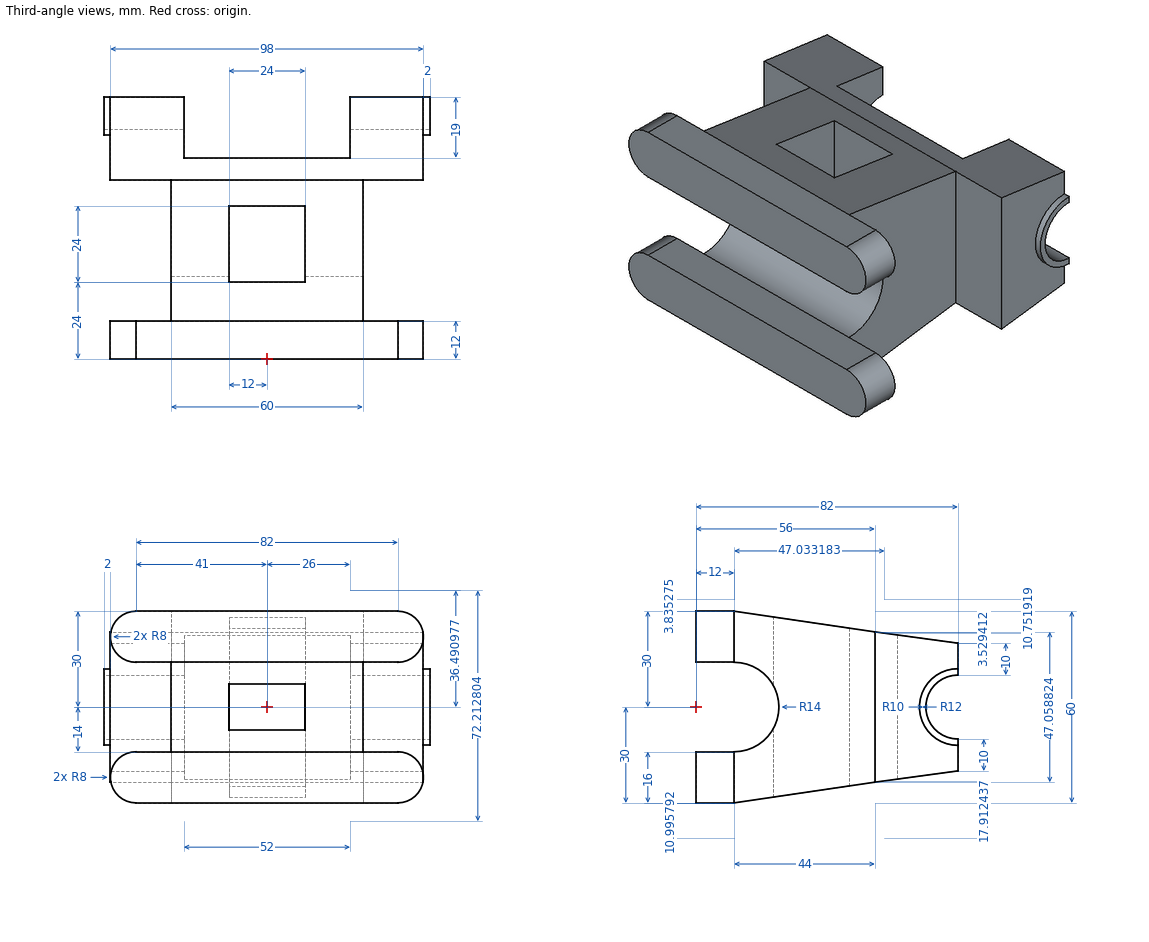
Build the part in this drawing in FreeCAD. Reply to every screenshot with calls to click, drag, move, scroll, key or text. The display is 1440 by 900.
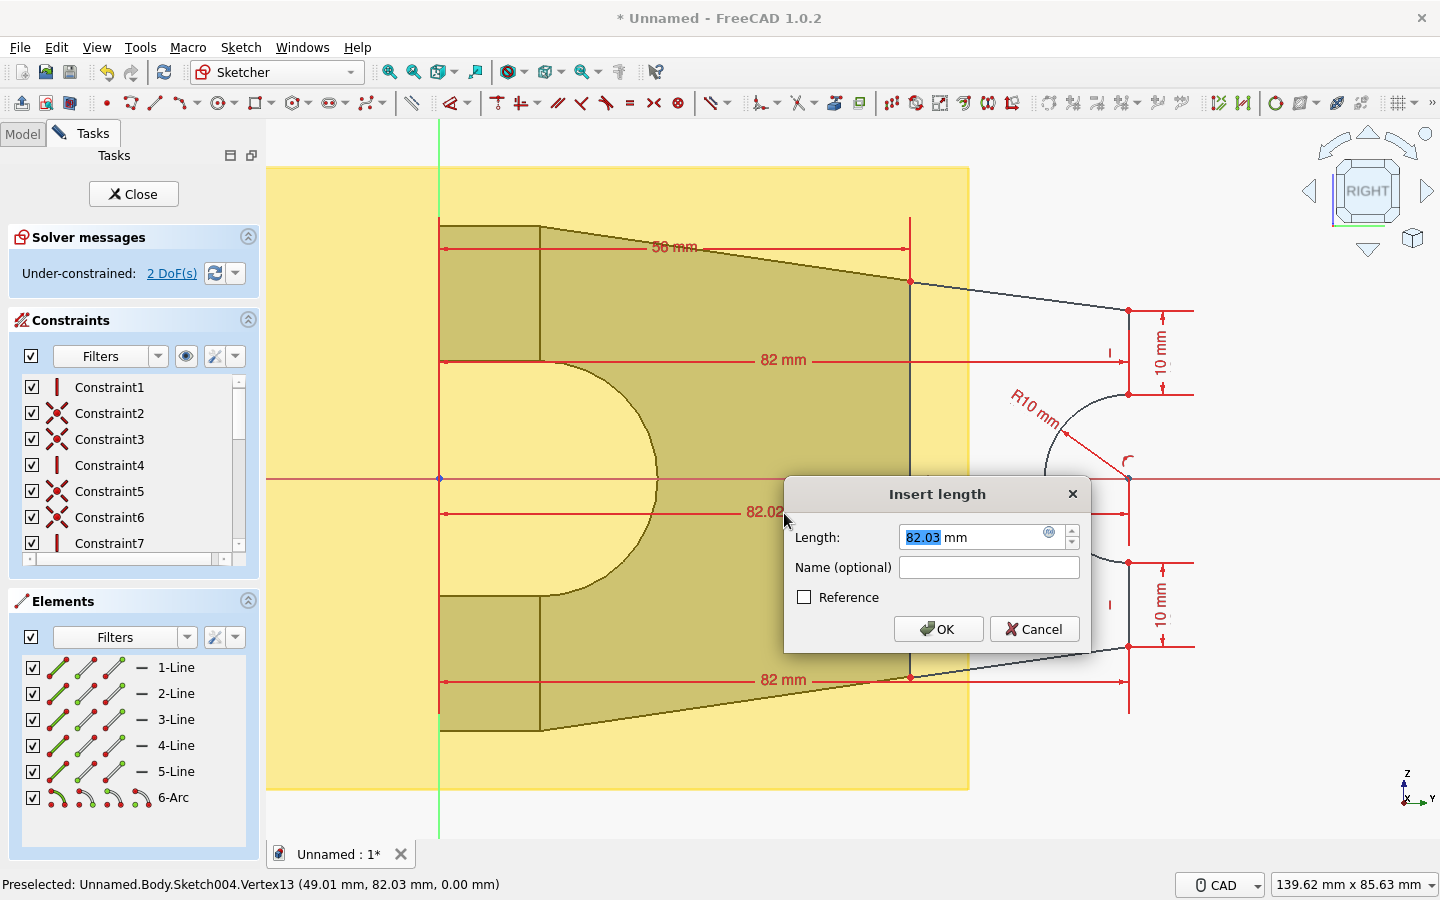
text(82)
key(Return)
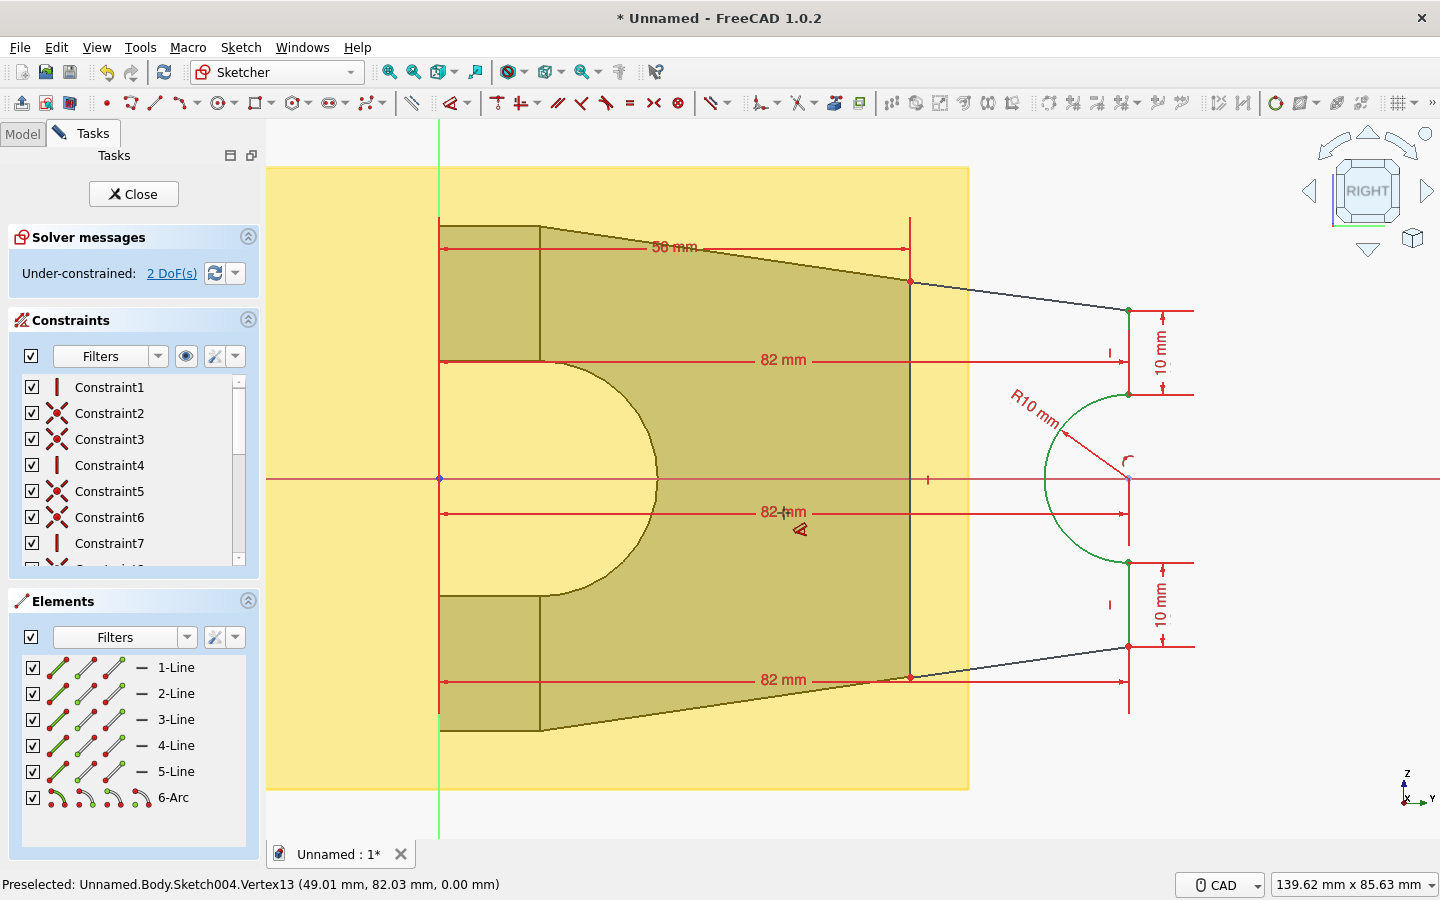
click(910, 401)
click(944, 389)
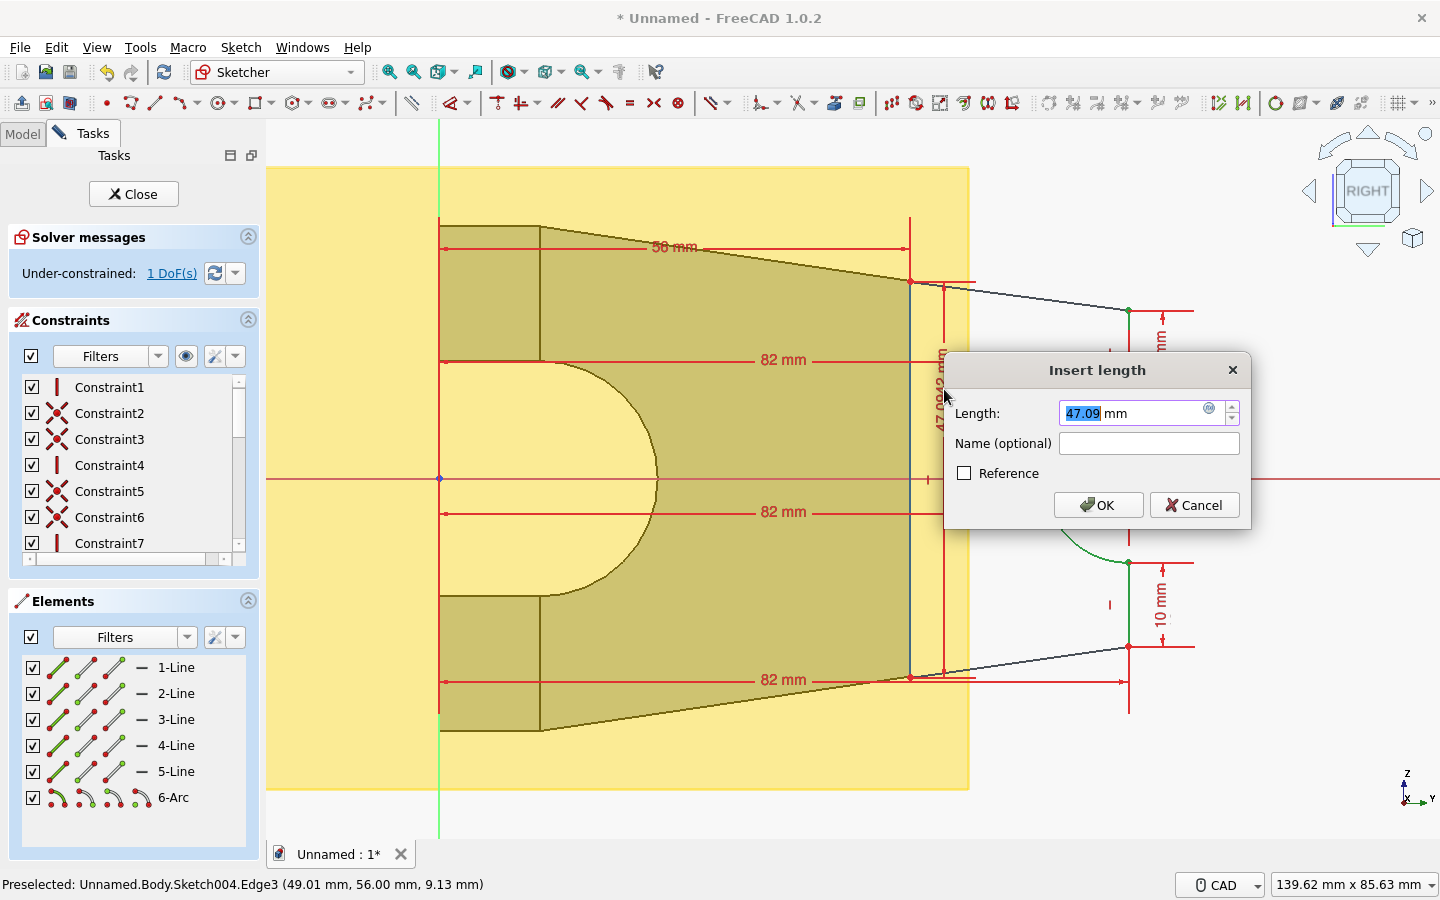
text(47.058824)
key(Return)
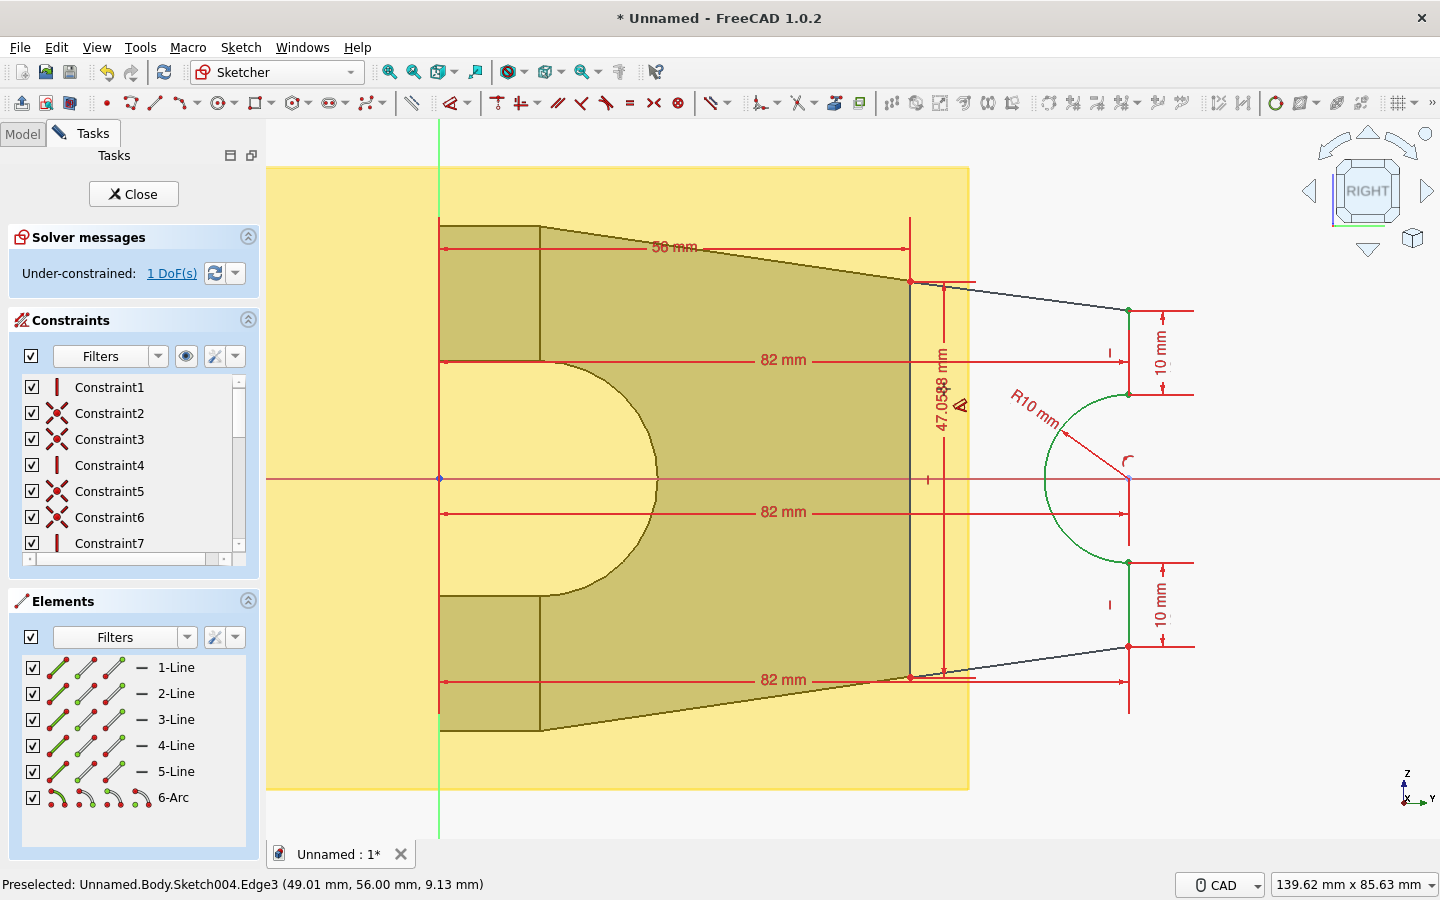
scroll(1063, 302, up, 2)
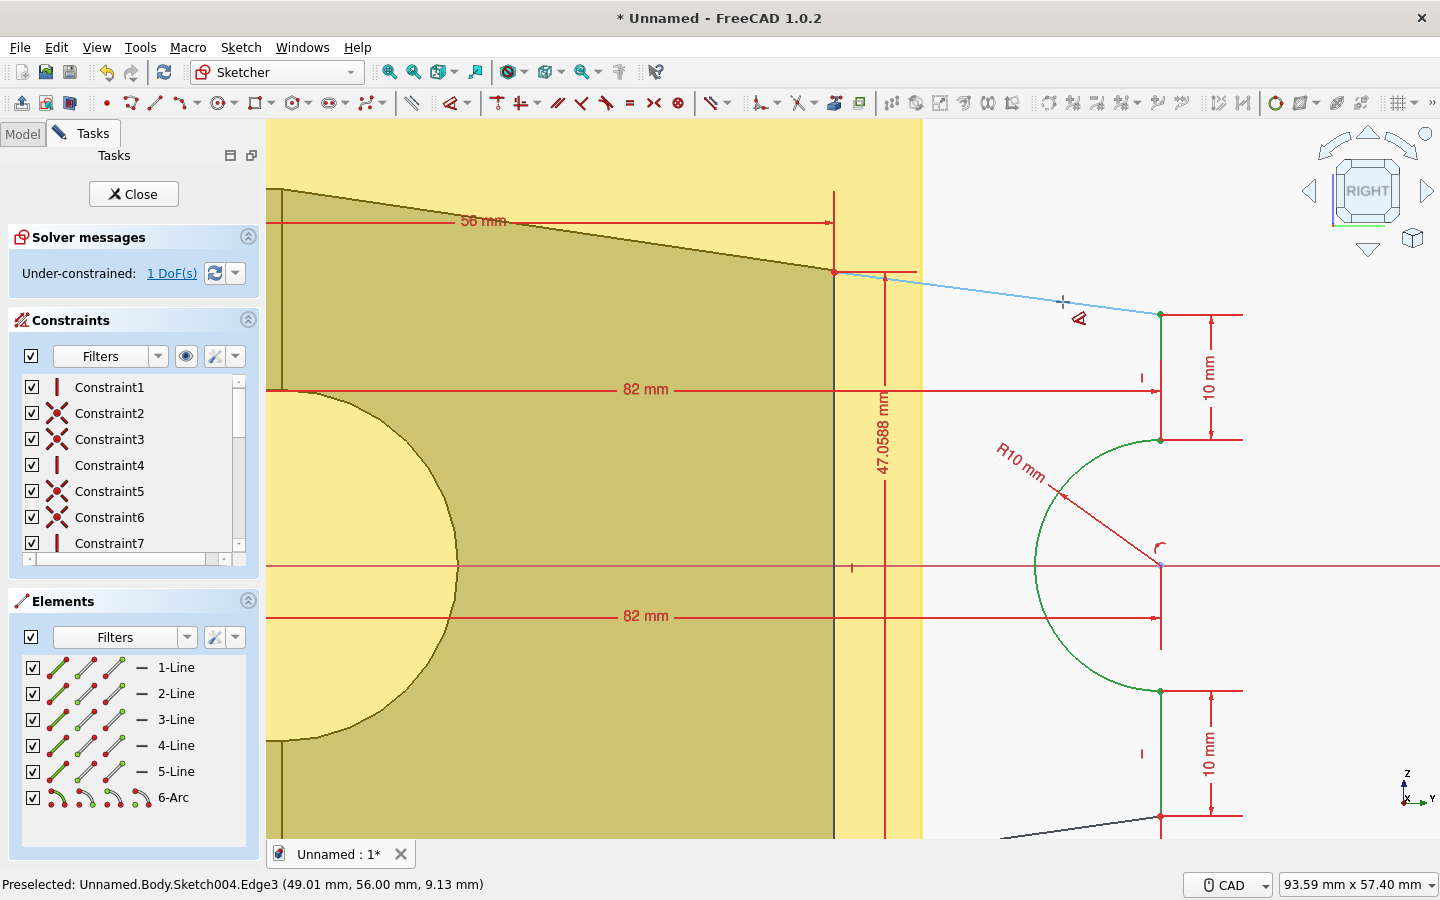
click(1063, 302)
click(1195, 293)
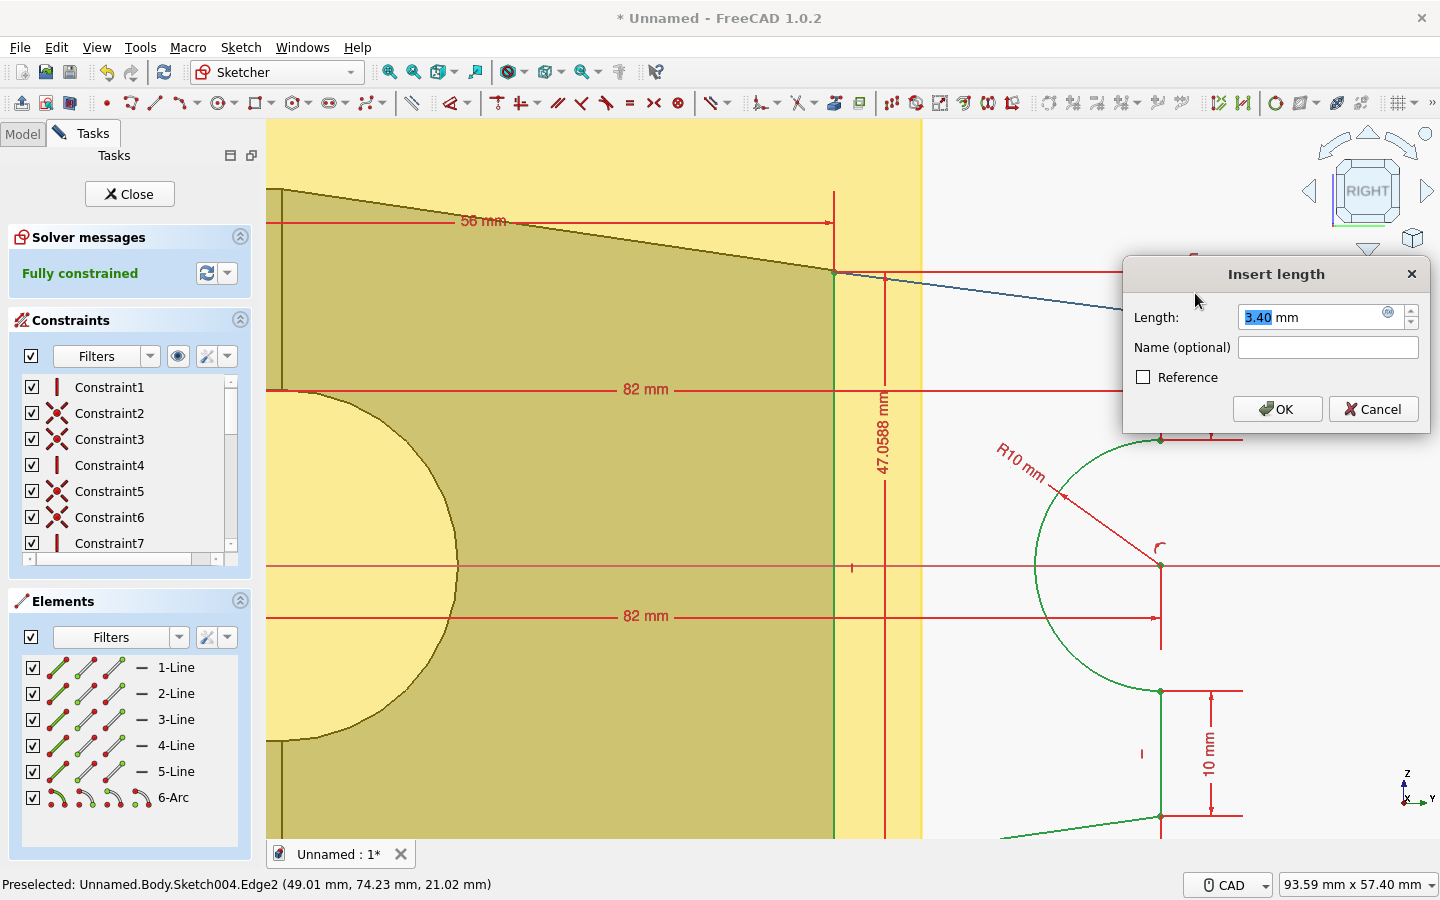
text(3.529412)
key(Return)
key(Escape)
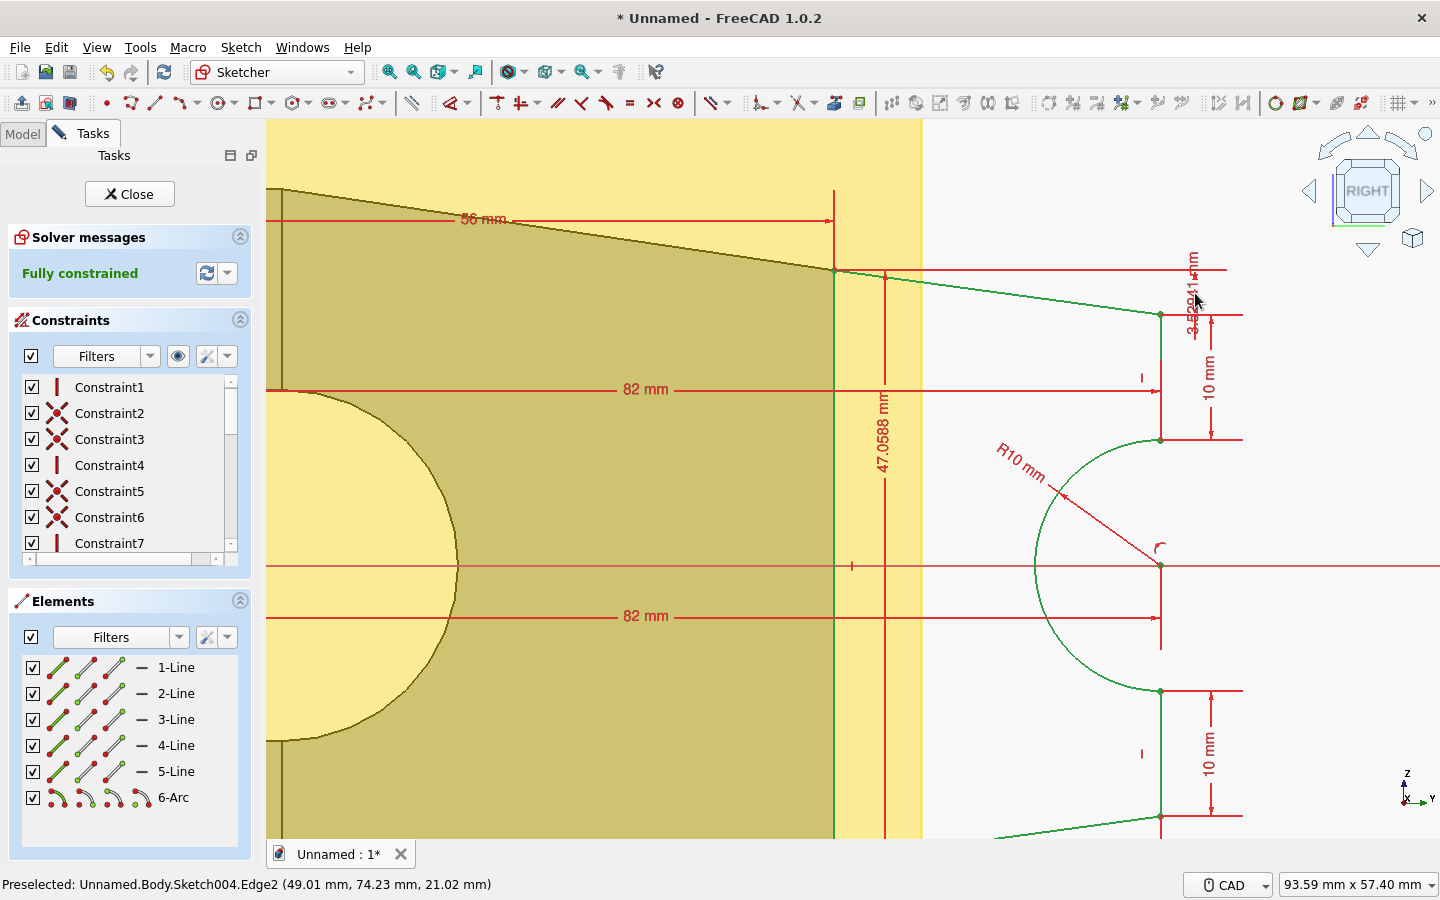
click(130, 194)